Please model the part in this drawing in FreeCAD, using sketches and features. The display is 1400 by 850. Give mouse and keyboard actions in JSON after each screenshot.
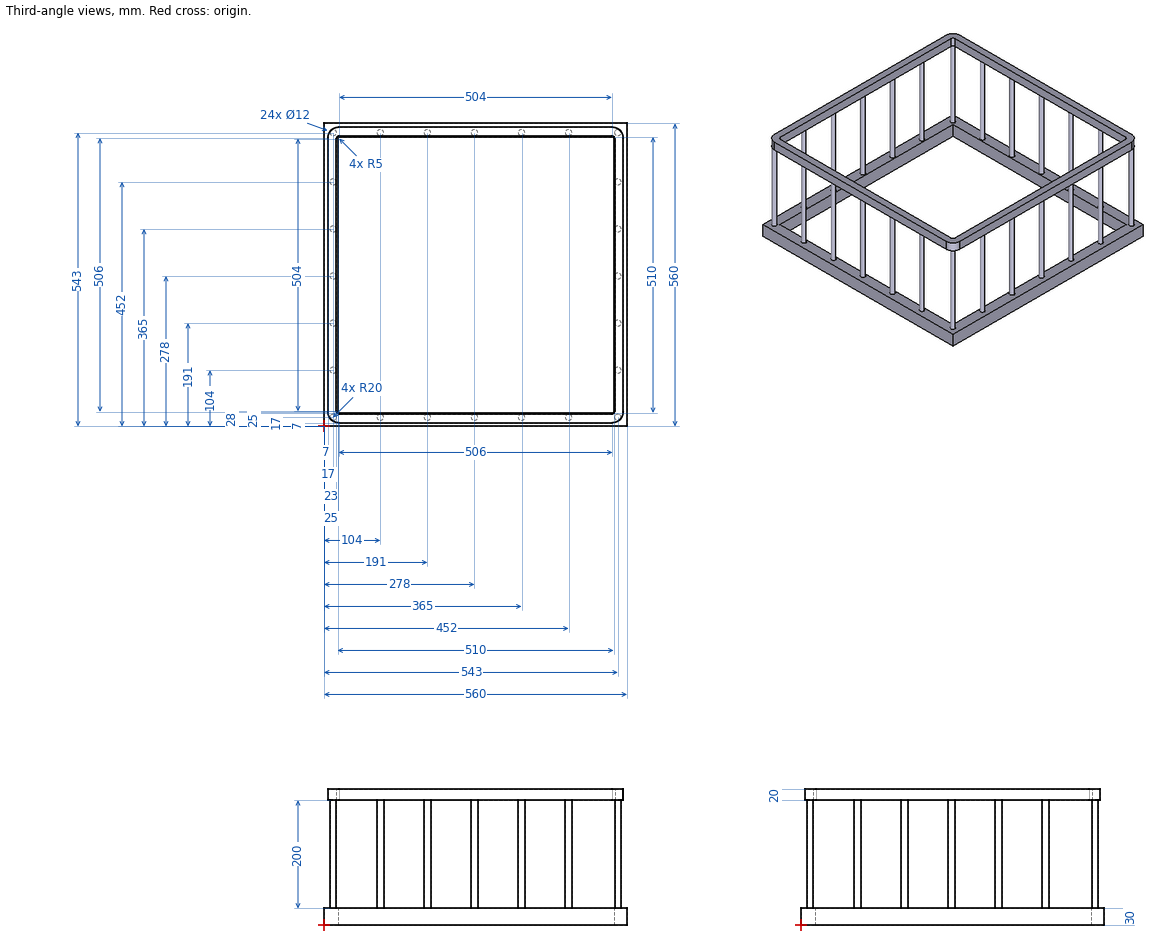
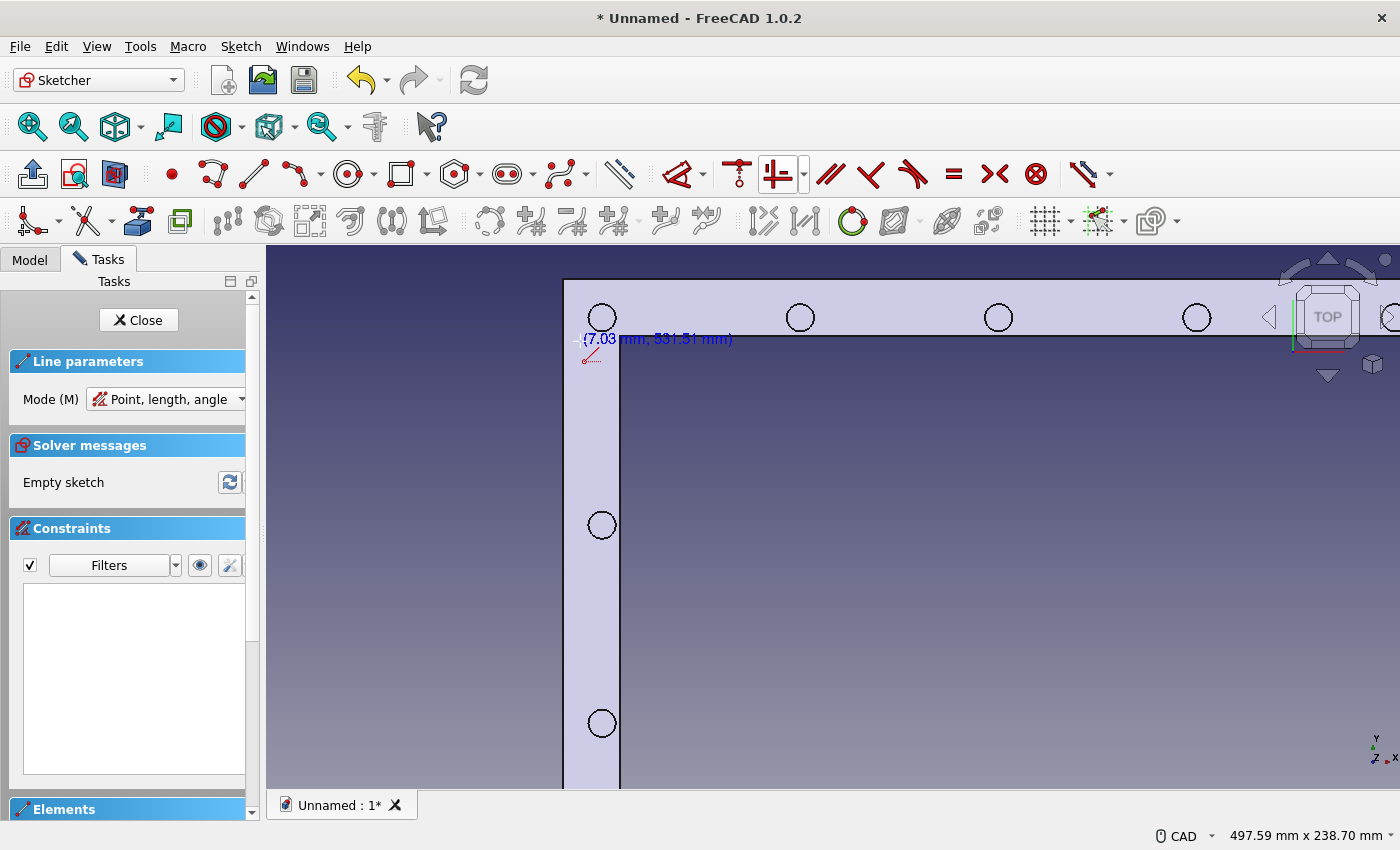
{"action": "left_click", "coordinate": [579, 341]}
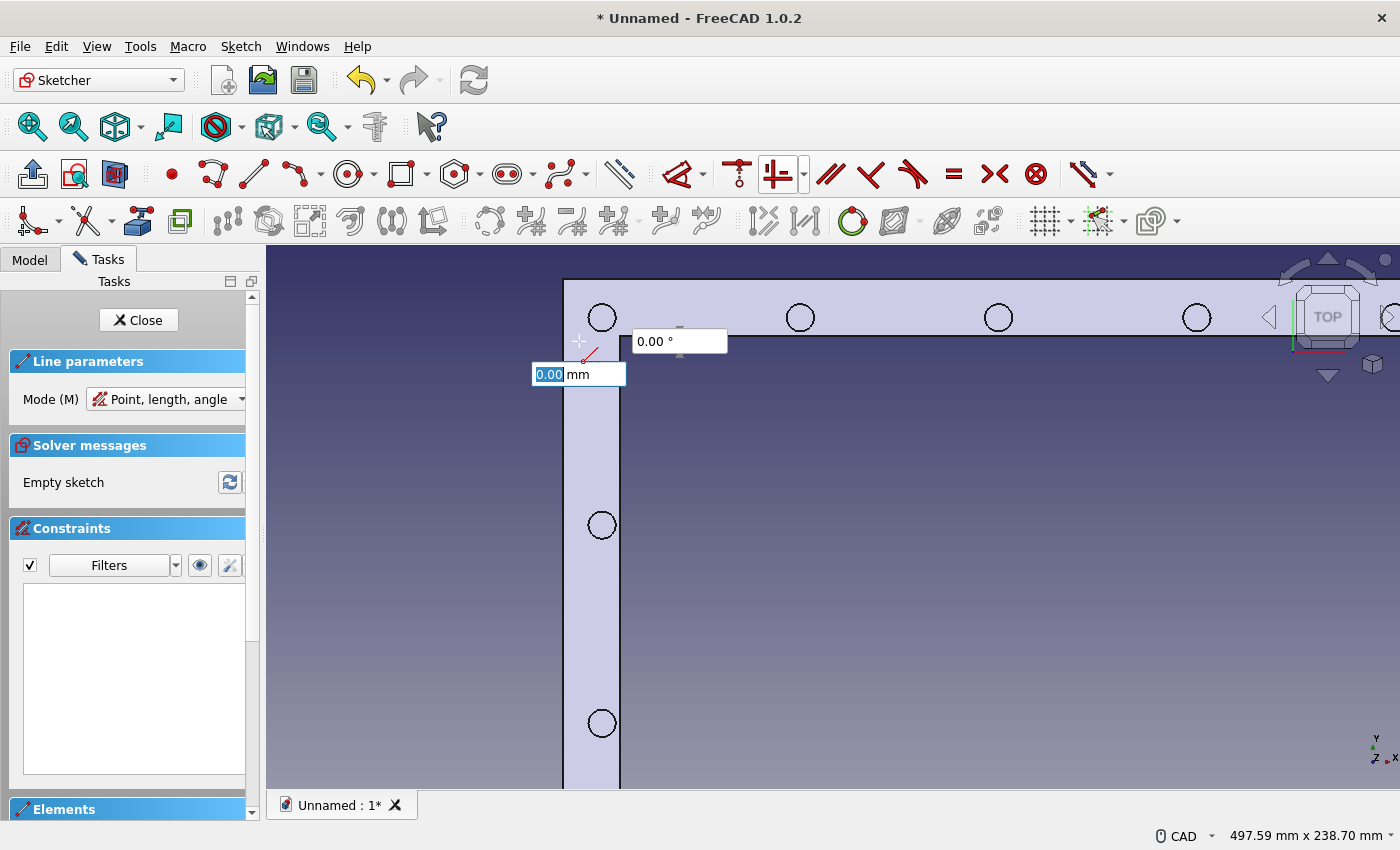
{"action": "scroll", "coordinate": [580, 341], "scroll_direction": "down", "scroll_amount": 6}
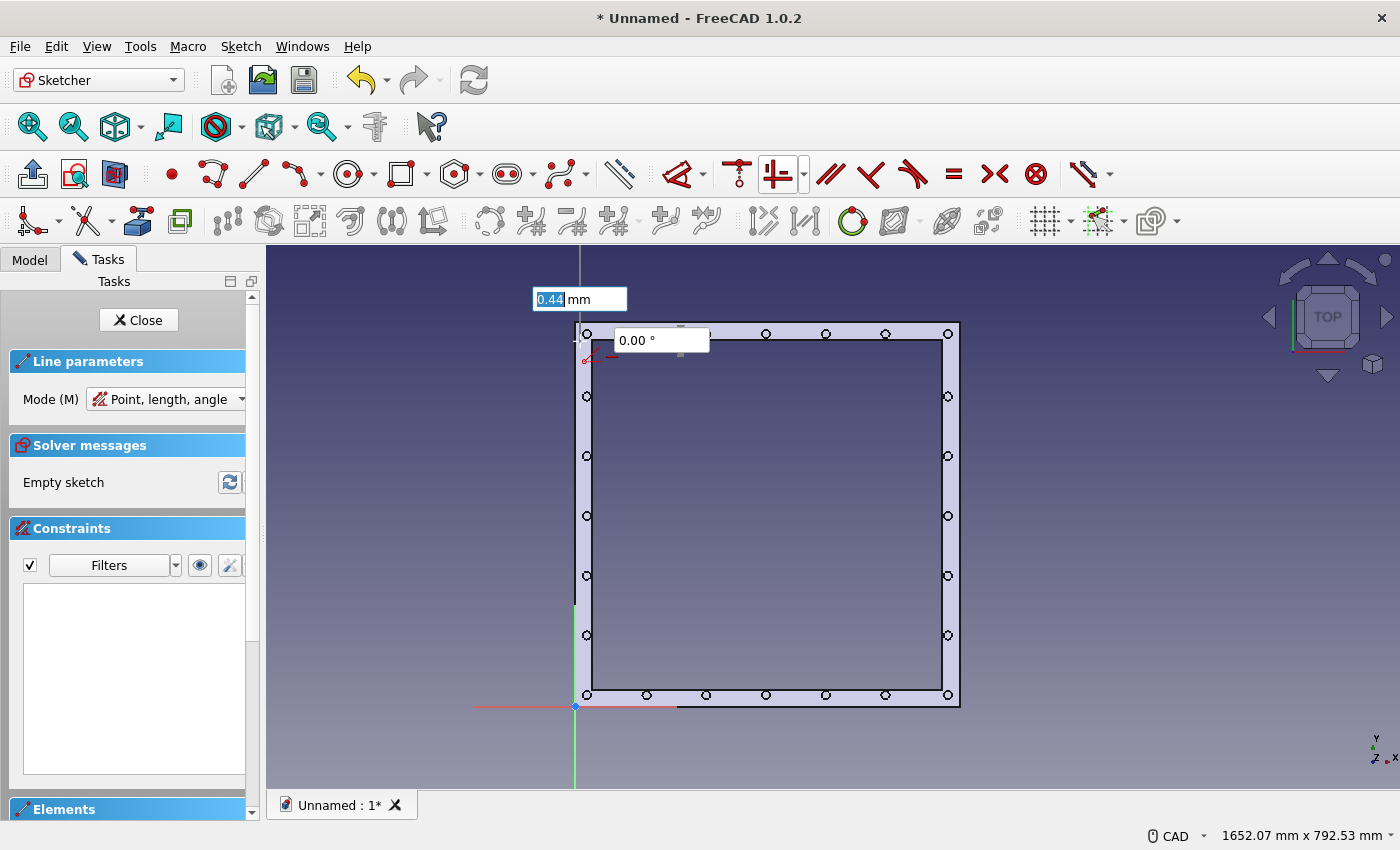
{"action": "scroll", "coordinate": [580, 688], "scroll_direction": "up", "scroll_amount": 6}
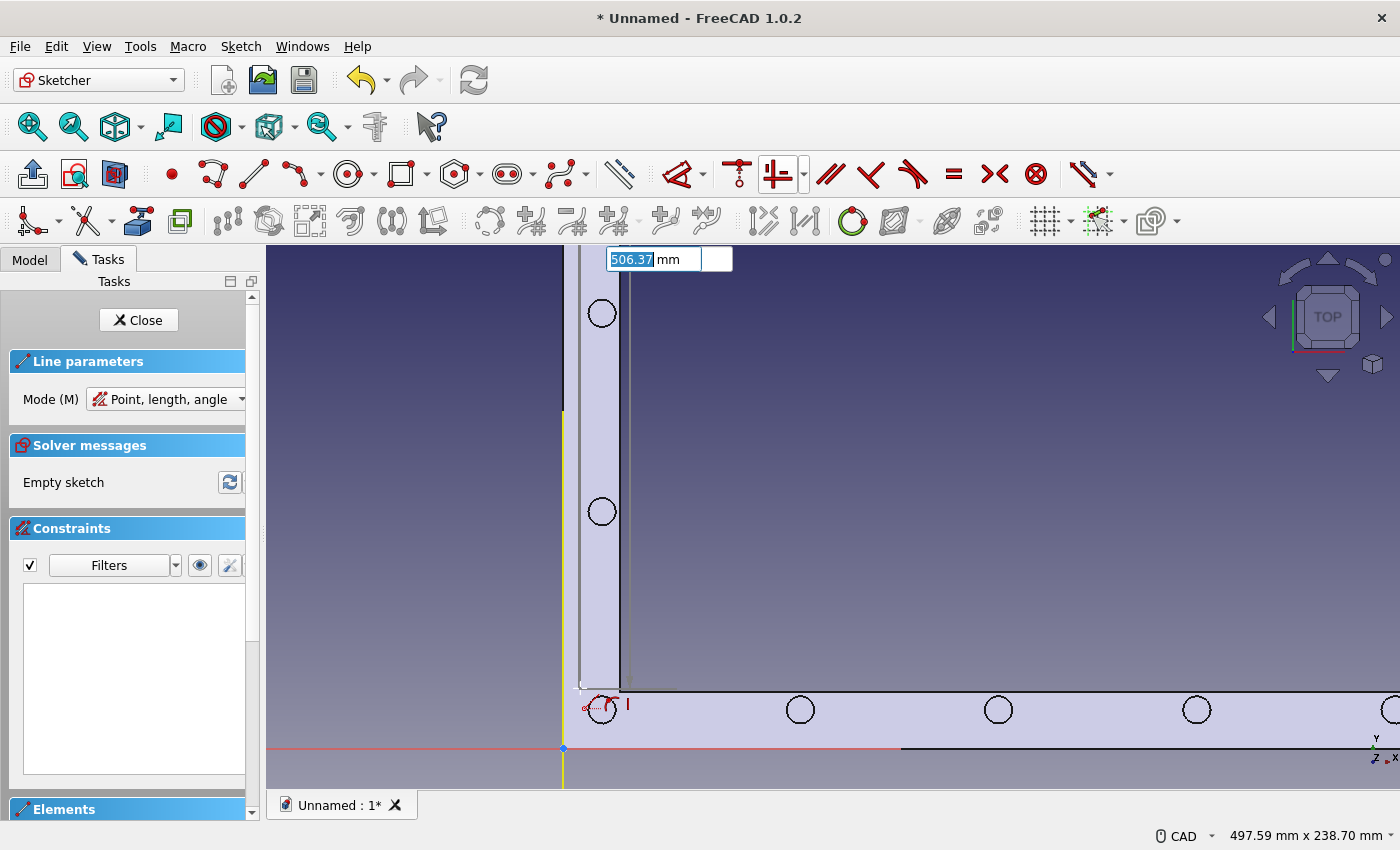
{"action": "left_click", "coordinate": [579, 687]}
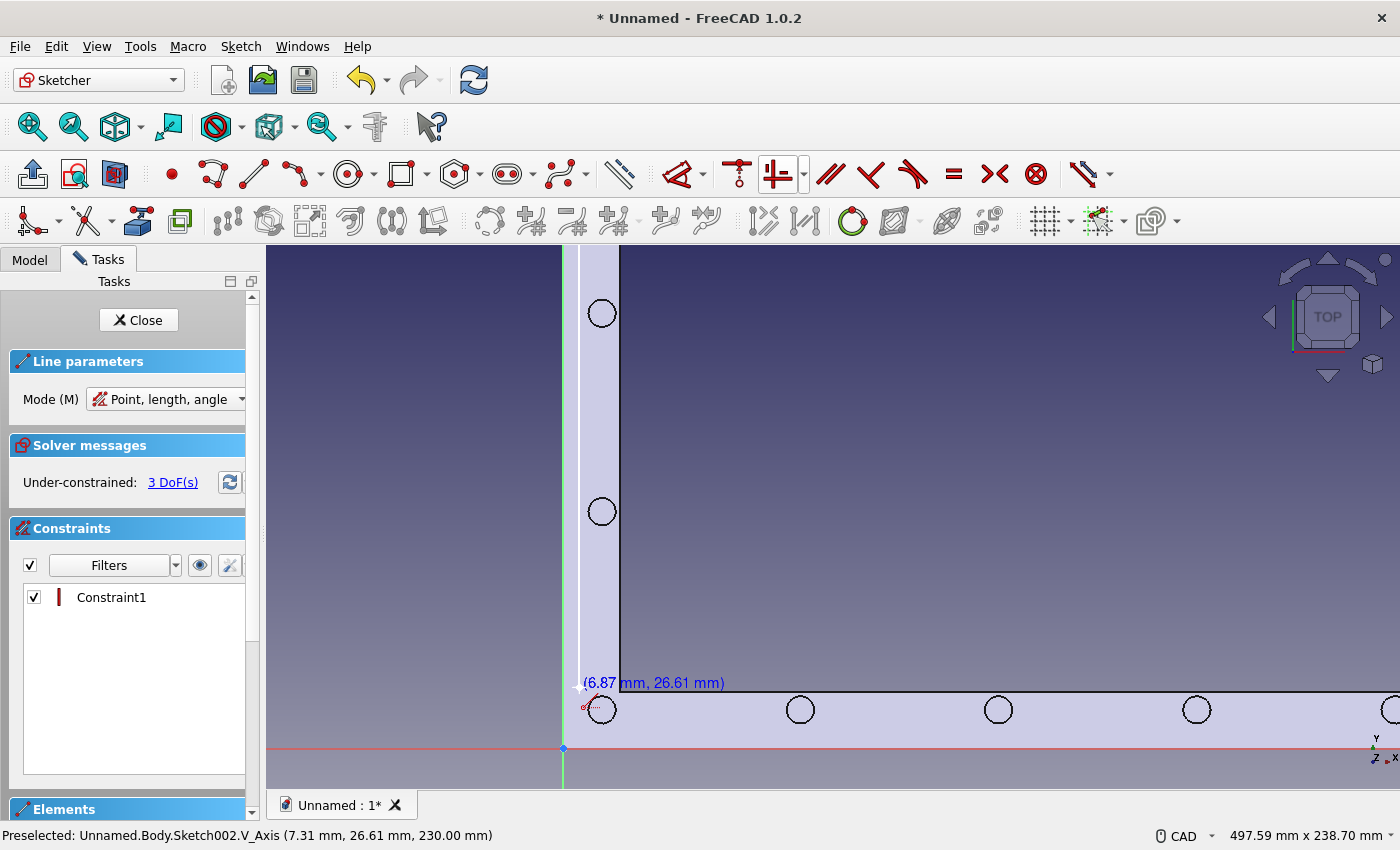
{"action": "left_click", "coordinate": [625, 733]}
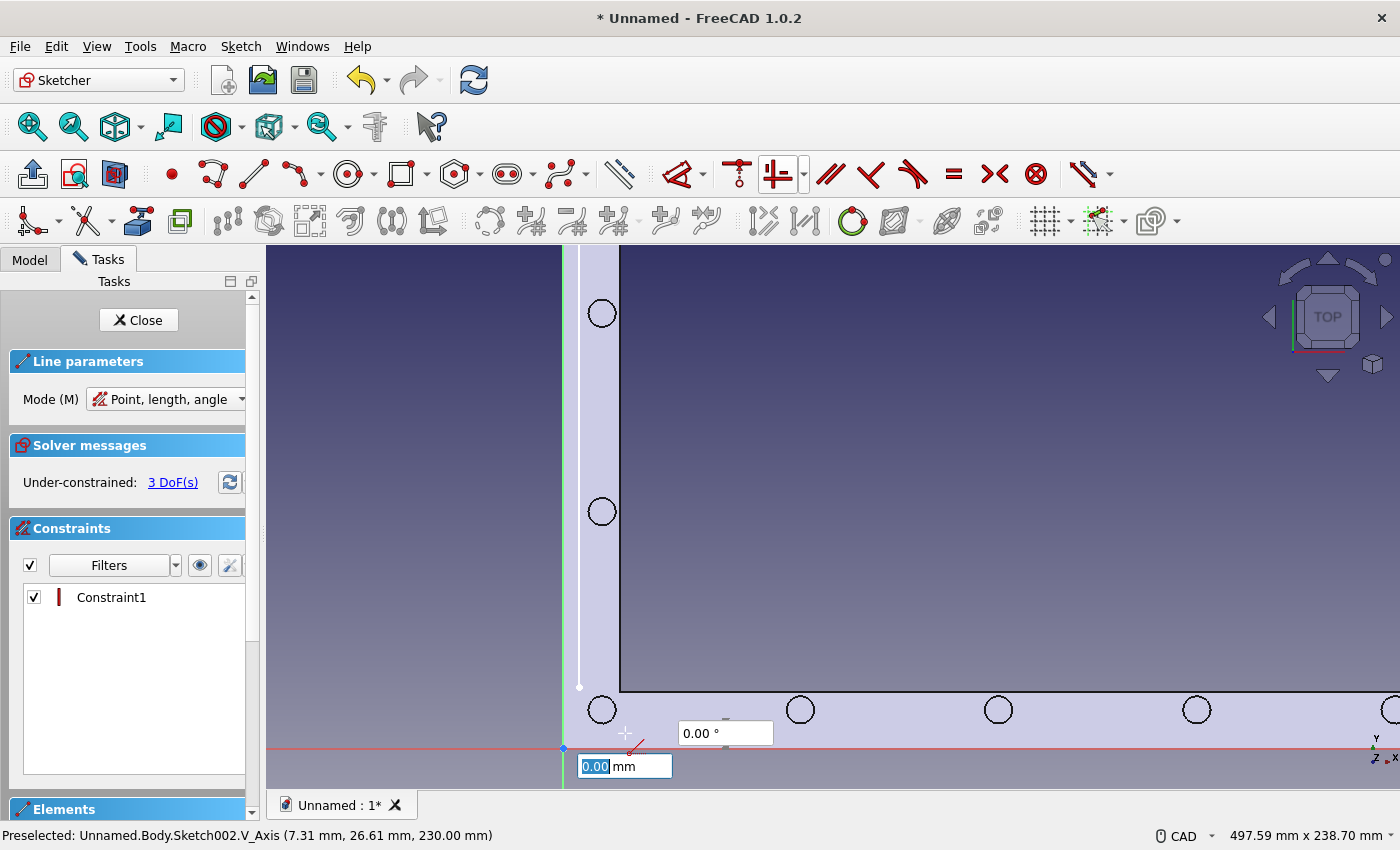
{"action": "scroll", "coordinate": [580, 689], "scroll_direction": "down", "scroll_amount": 6}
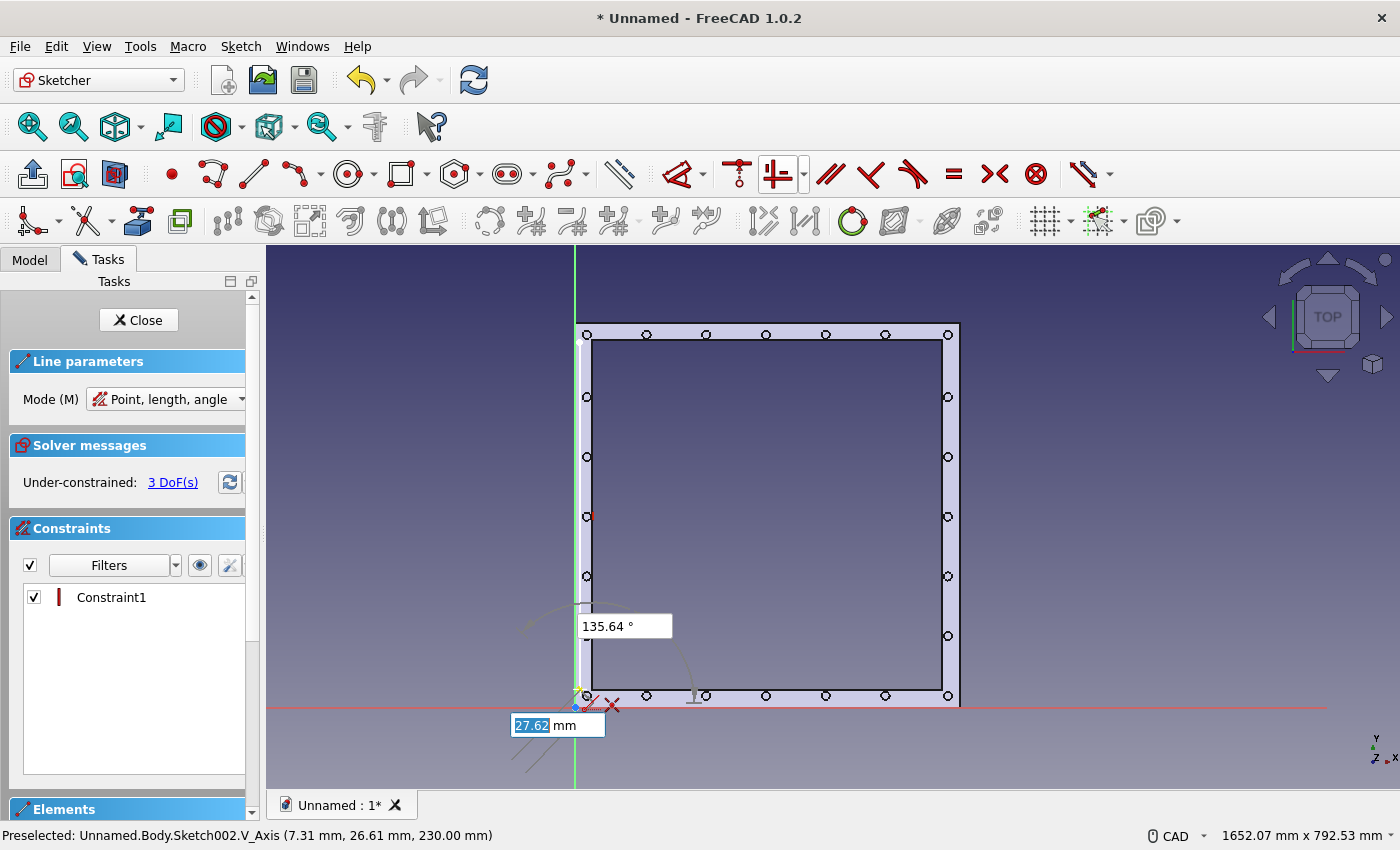
{"action": "scroll", "coordinate": [941, 703], "scroll_direction": "up", "scroll_amount": 6}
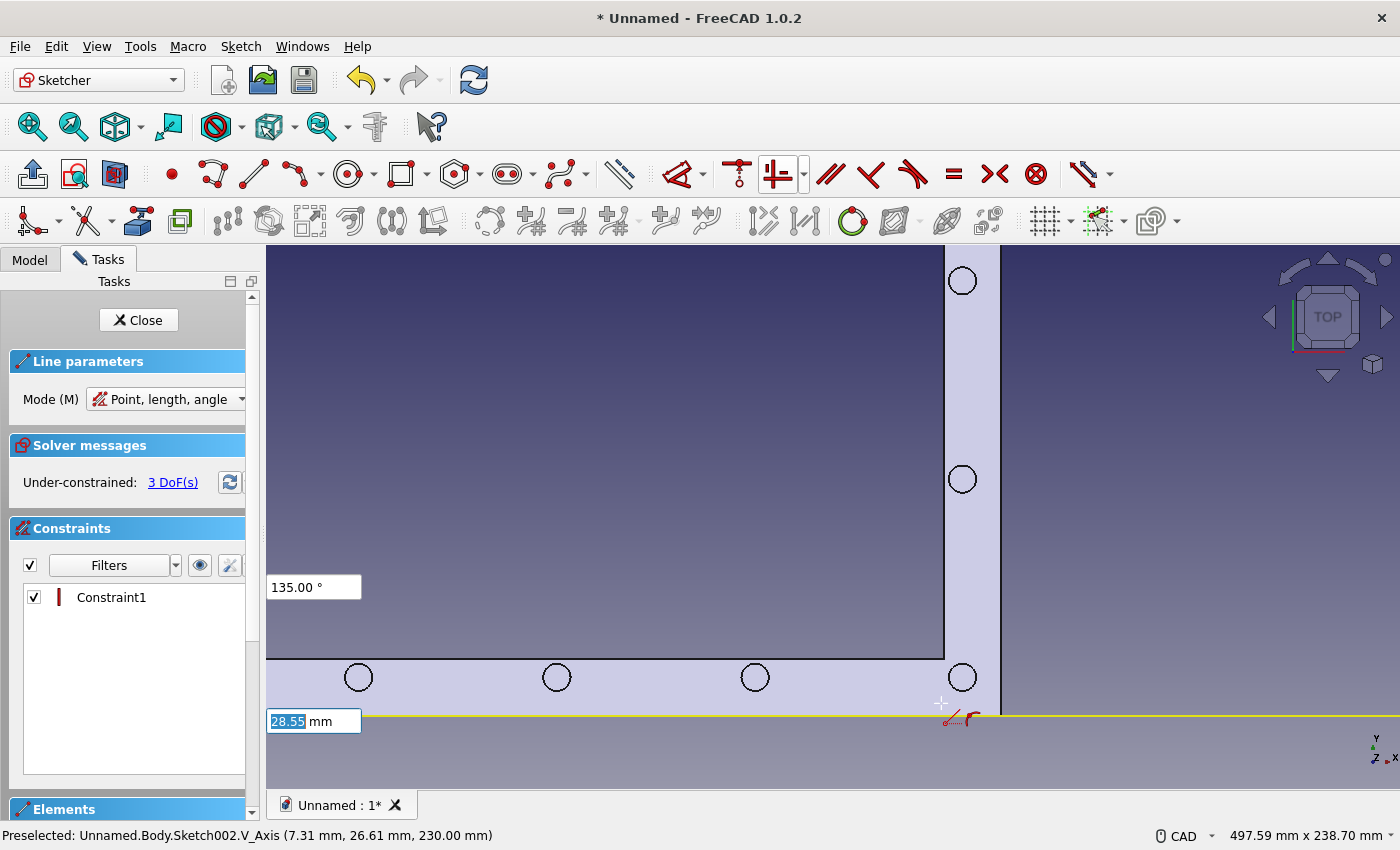
{"action": "left_click", "coordinate": [940, 700]}